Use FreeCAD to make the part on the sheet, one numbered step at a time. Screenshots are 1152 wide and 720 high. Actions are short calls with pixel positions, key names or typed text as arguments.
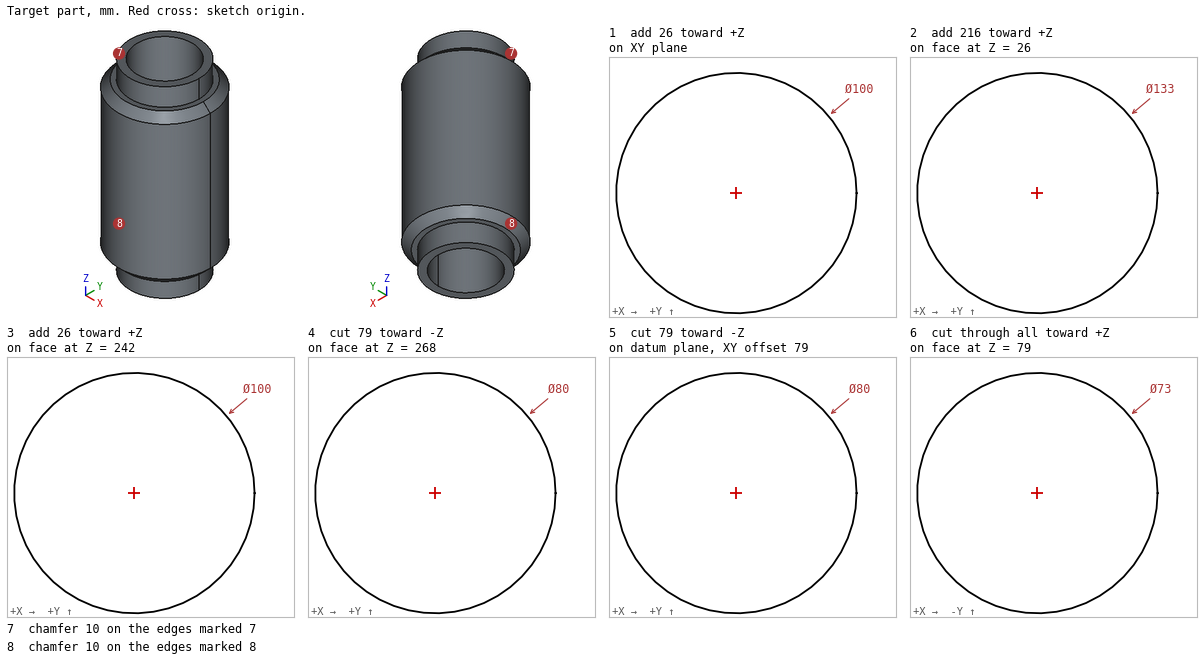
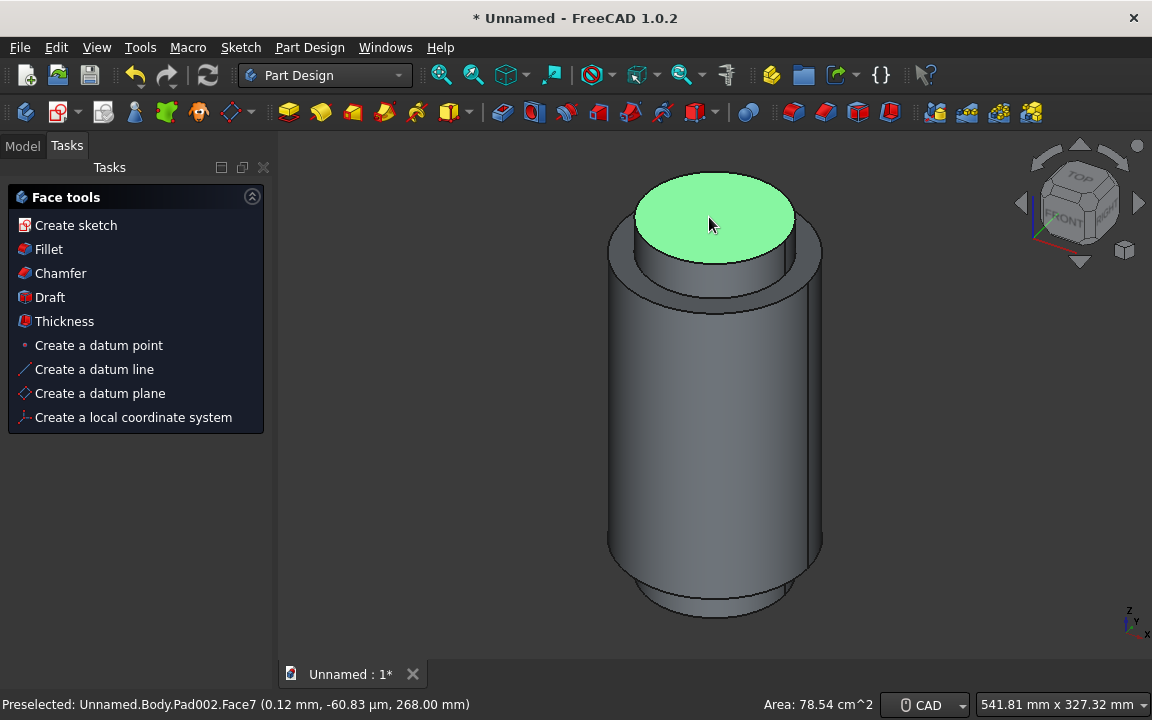
click(58, 112)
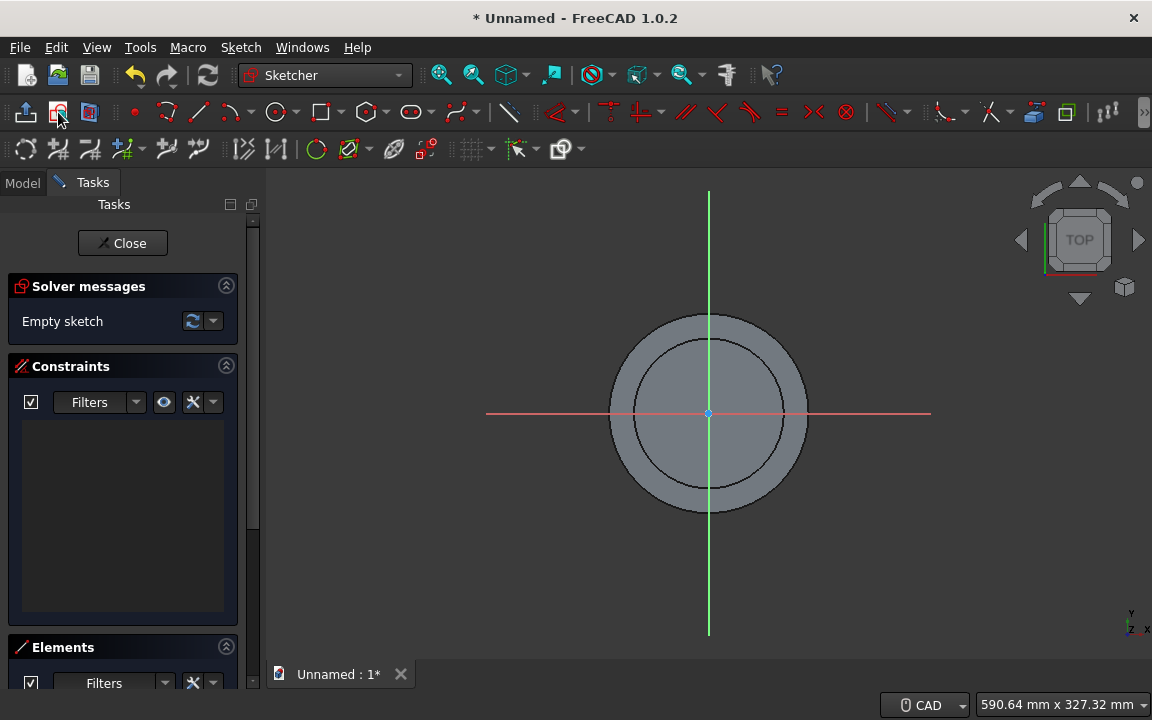
scroll(749, 414, up, 5)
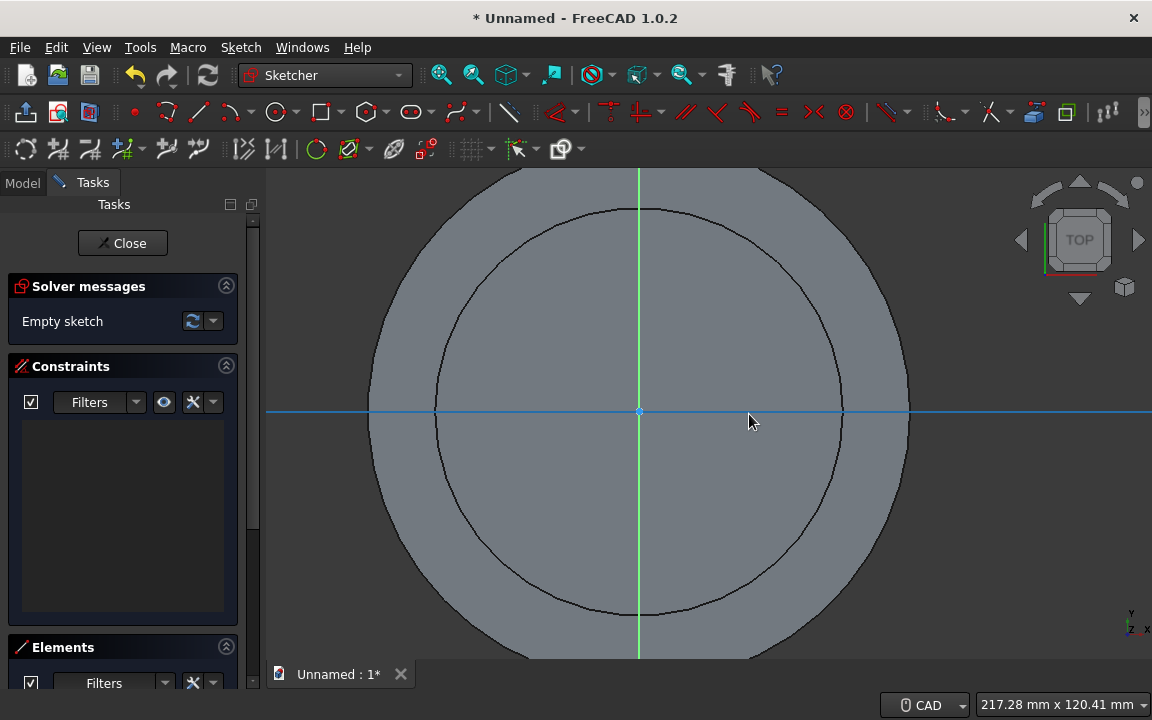
click(276, 112)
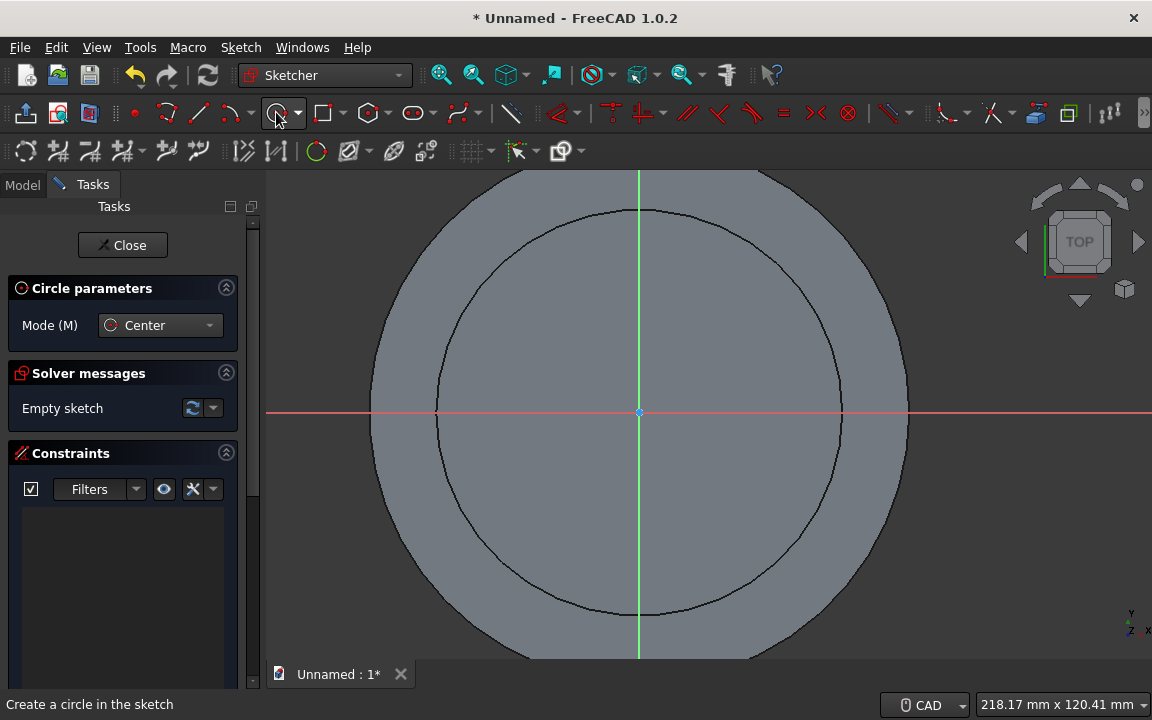
click(639, 413)
move(754, 298)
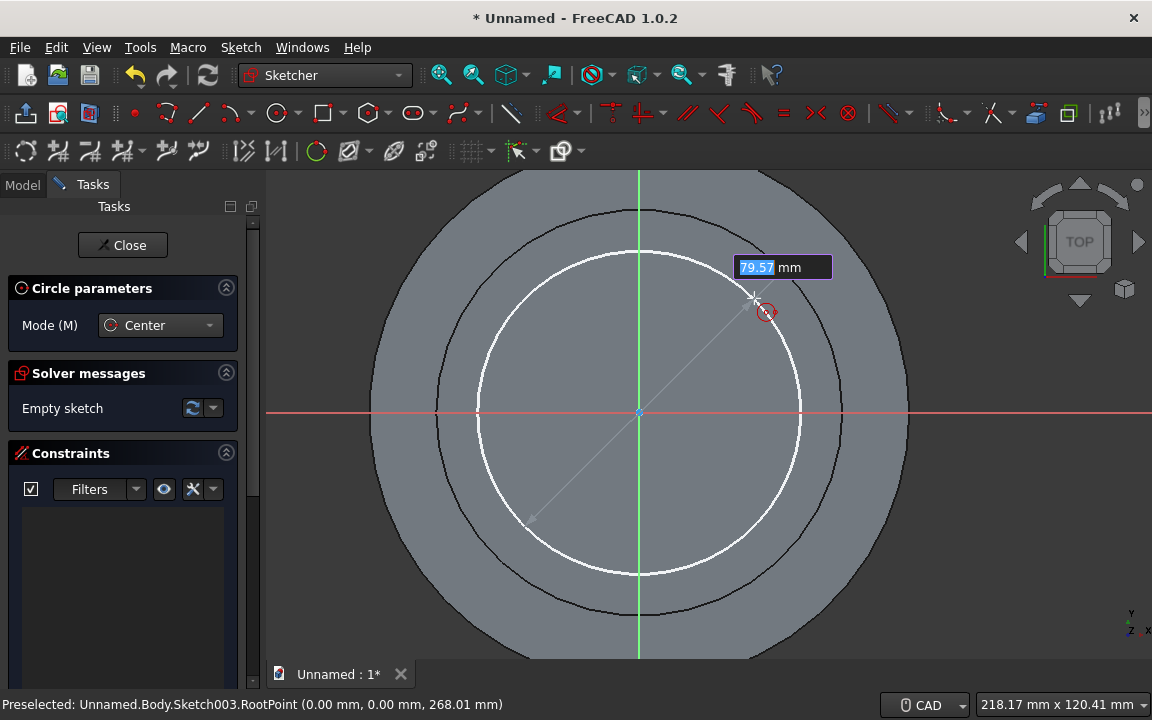
text(80)
key(Return)
key(Escape)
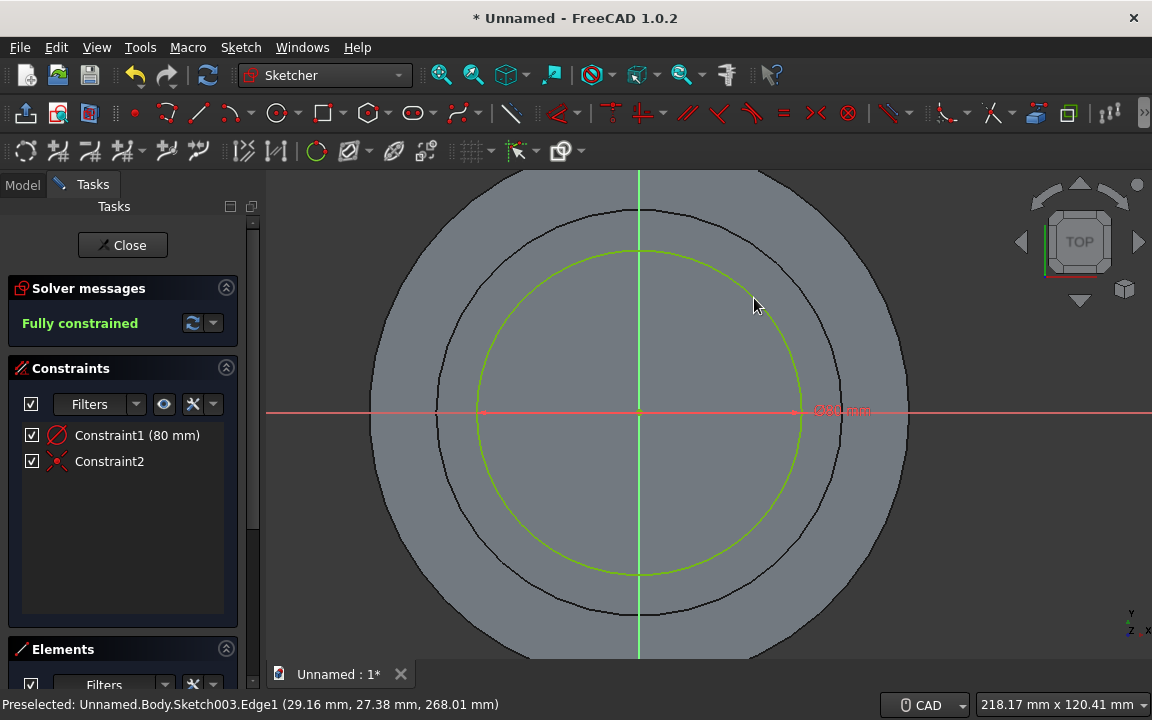
click(123, 245)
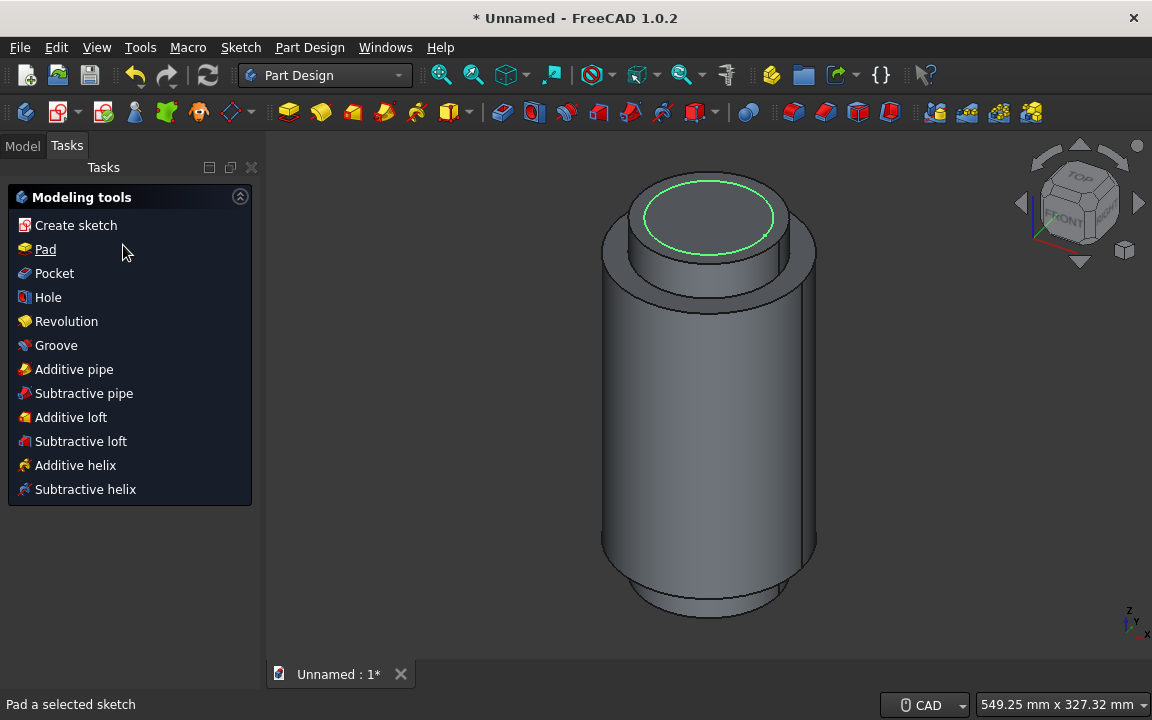
click(504, 112)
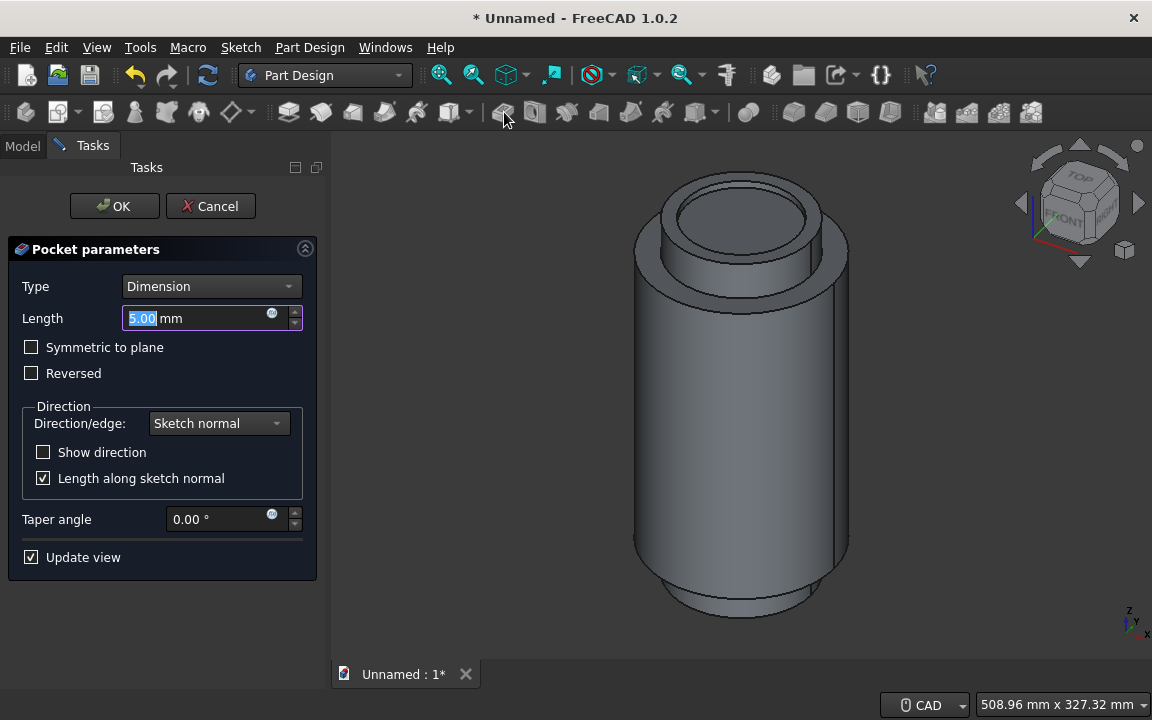
text(79)
key(Tab)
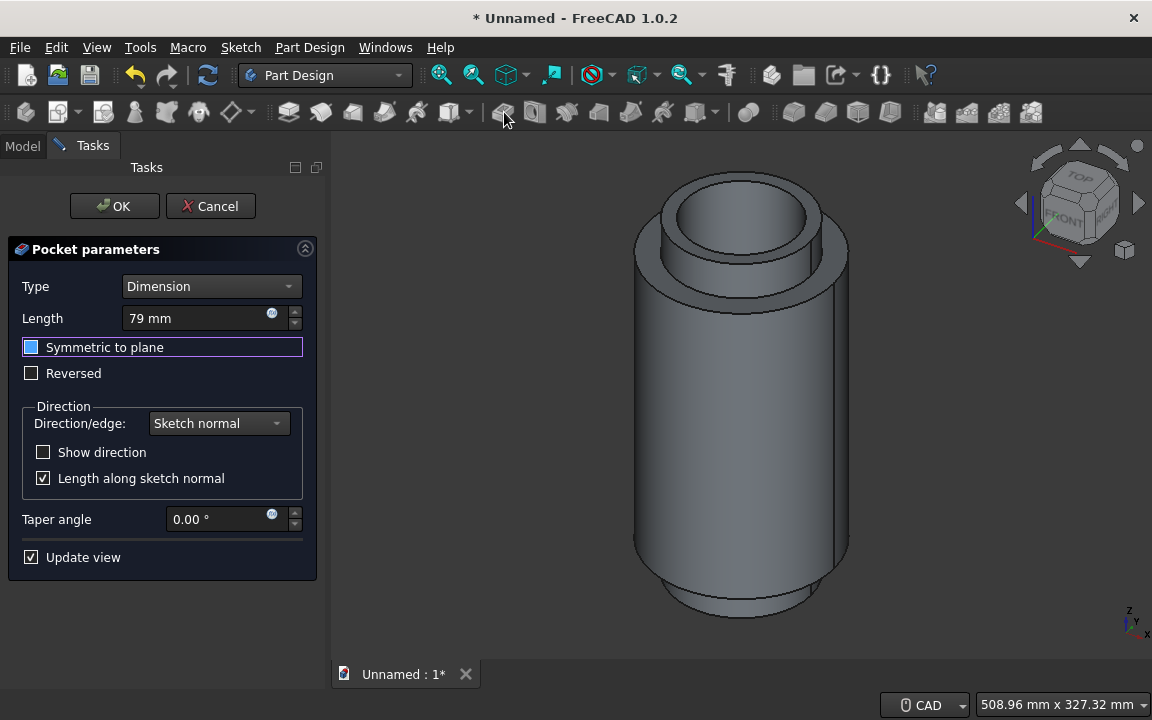
click(115, 206)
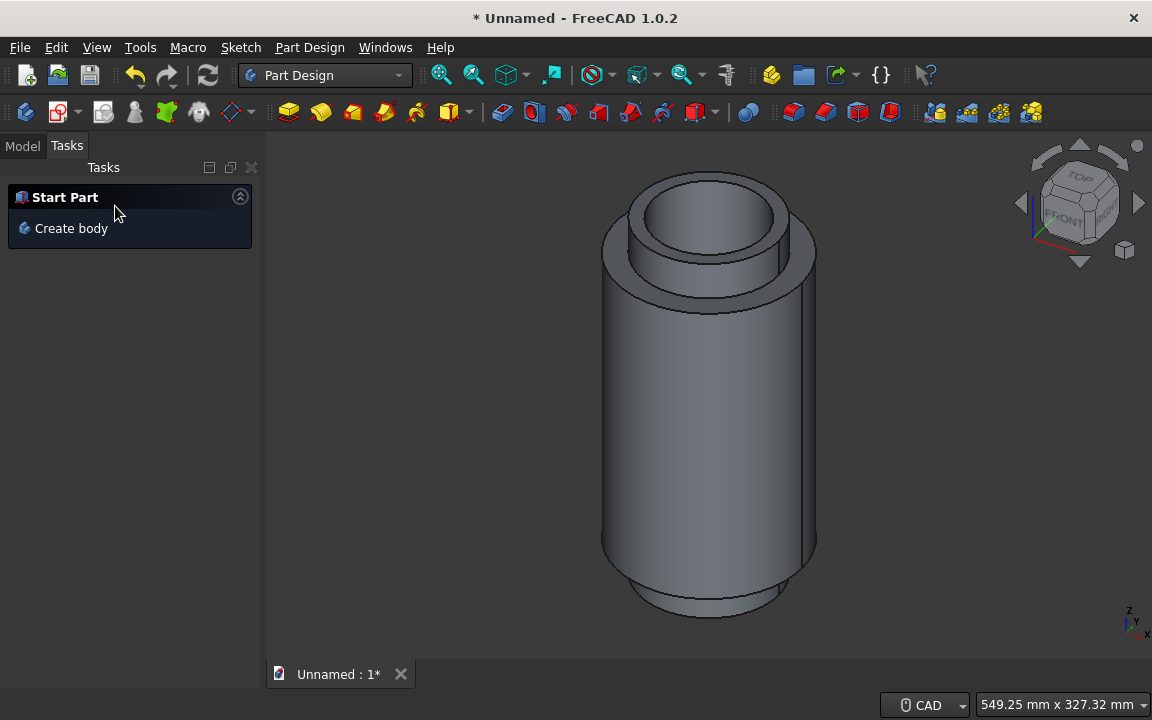
click(23, 145)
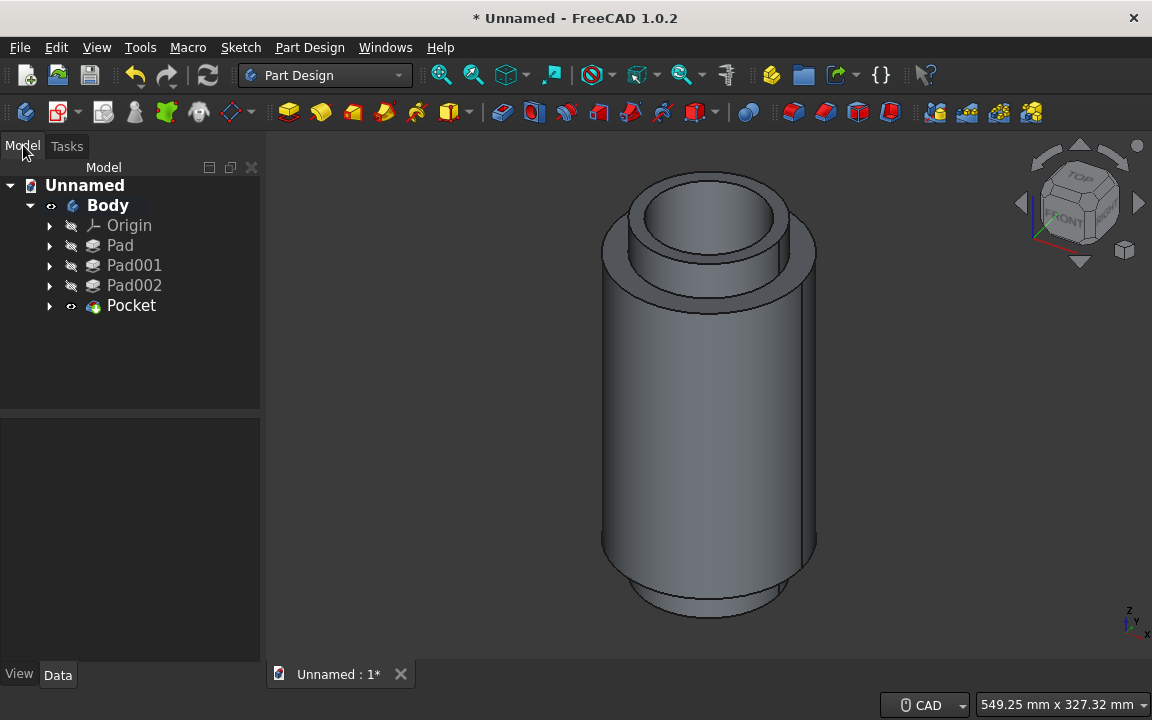
click(50, 226)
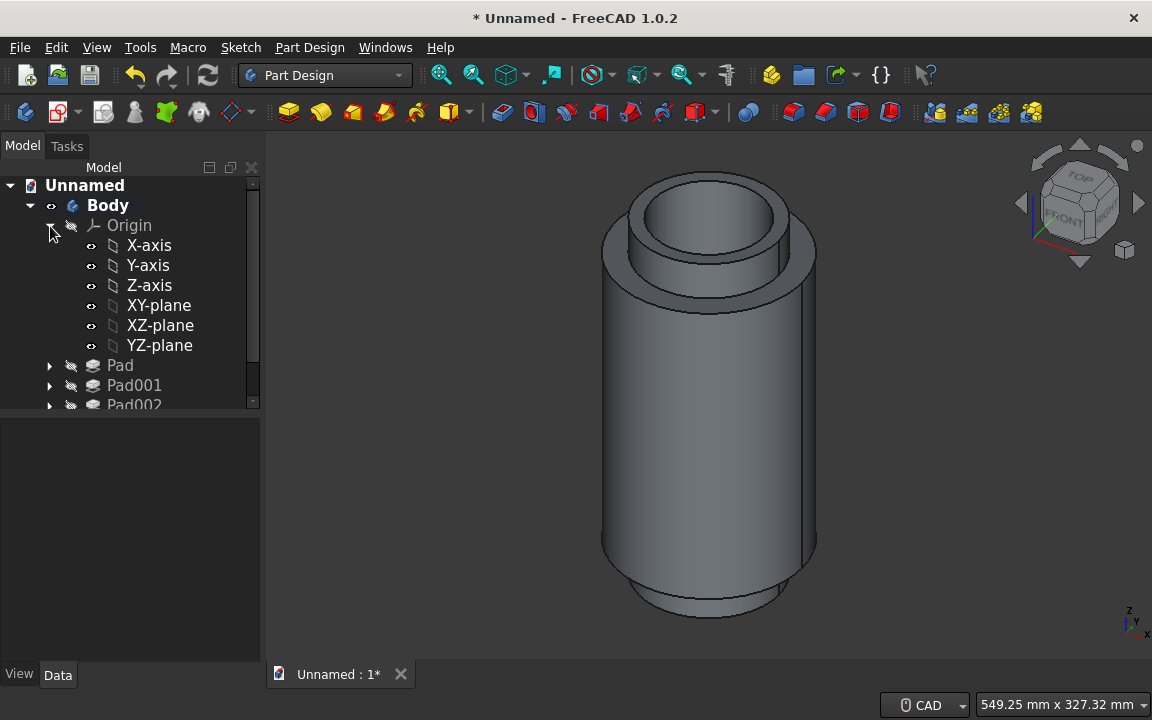
click(136, 306)